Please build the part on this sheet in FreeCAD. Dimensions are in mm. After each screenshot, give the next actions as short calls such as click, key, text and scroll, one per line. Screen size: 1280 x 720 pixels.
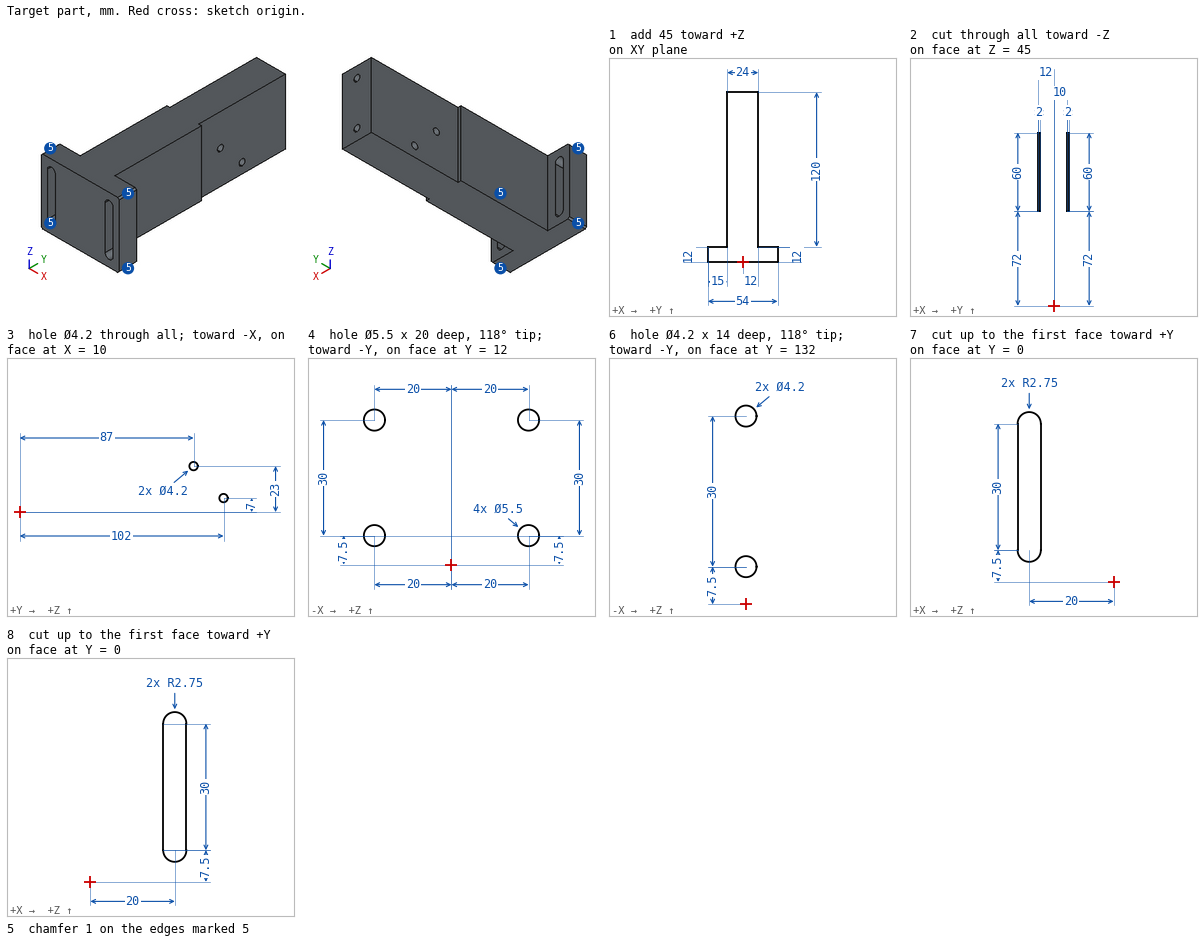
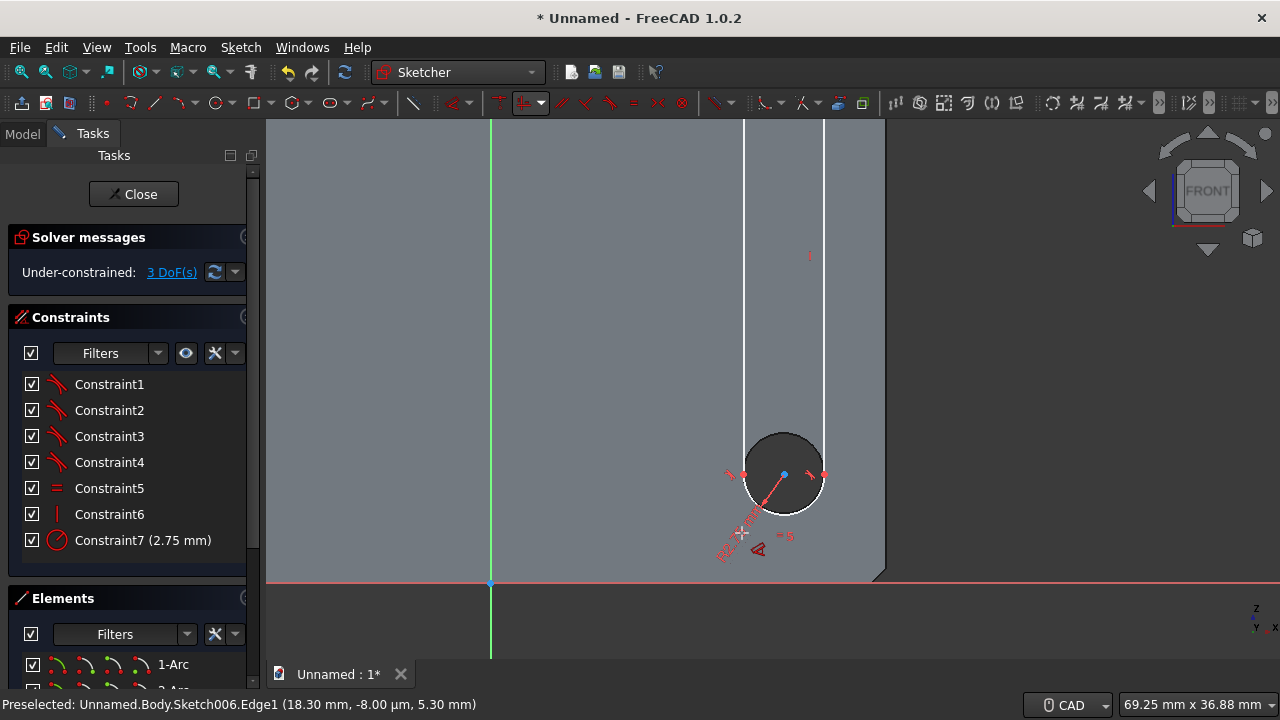
click(744, 343)
click(778, 311)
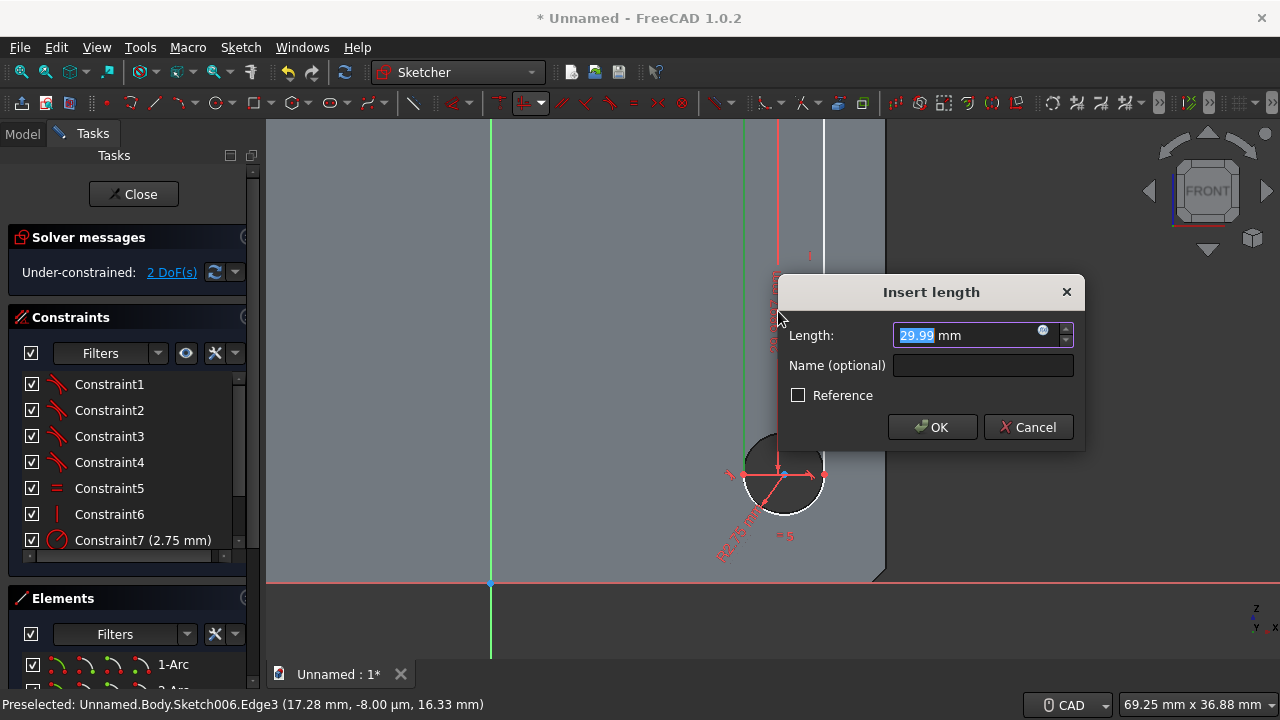
text(30)
key(Return)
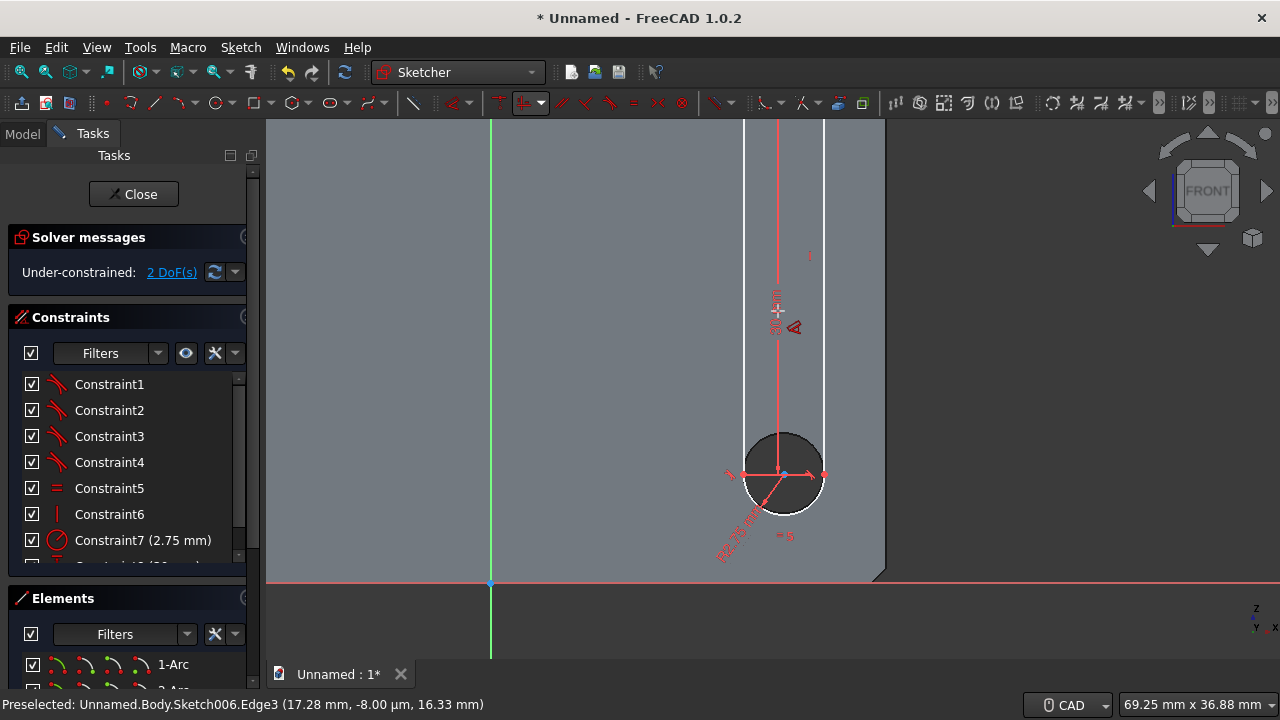
click(784, 475)
click(637, 617)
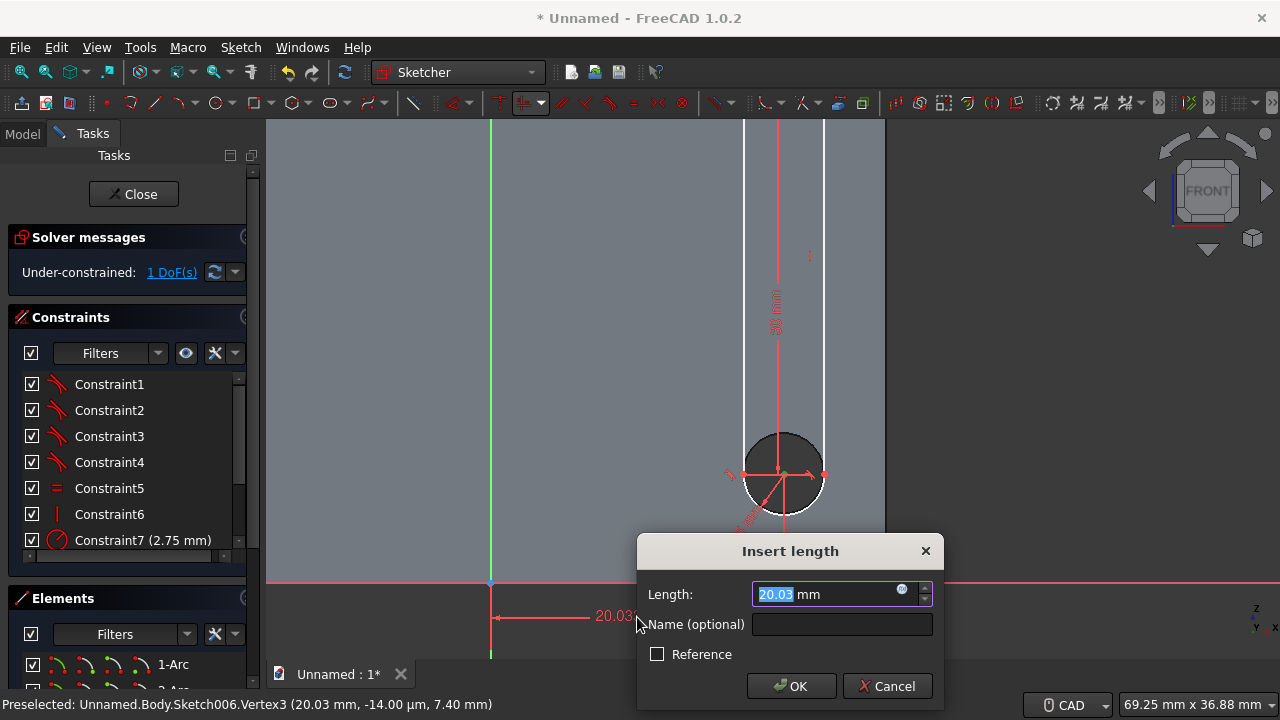
text(20)
key(Return)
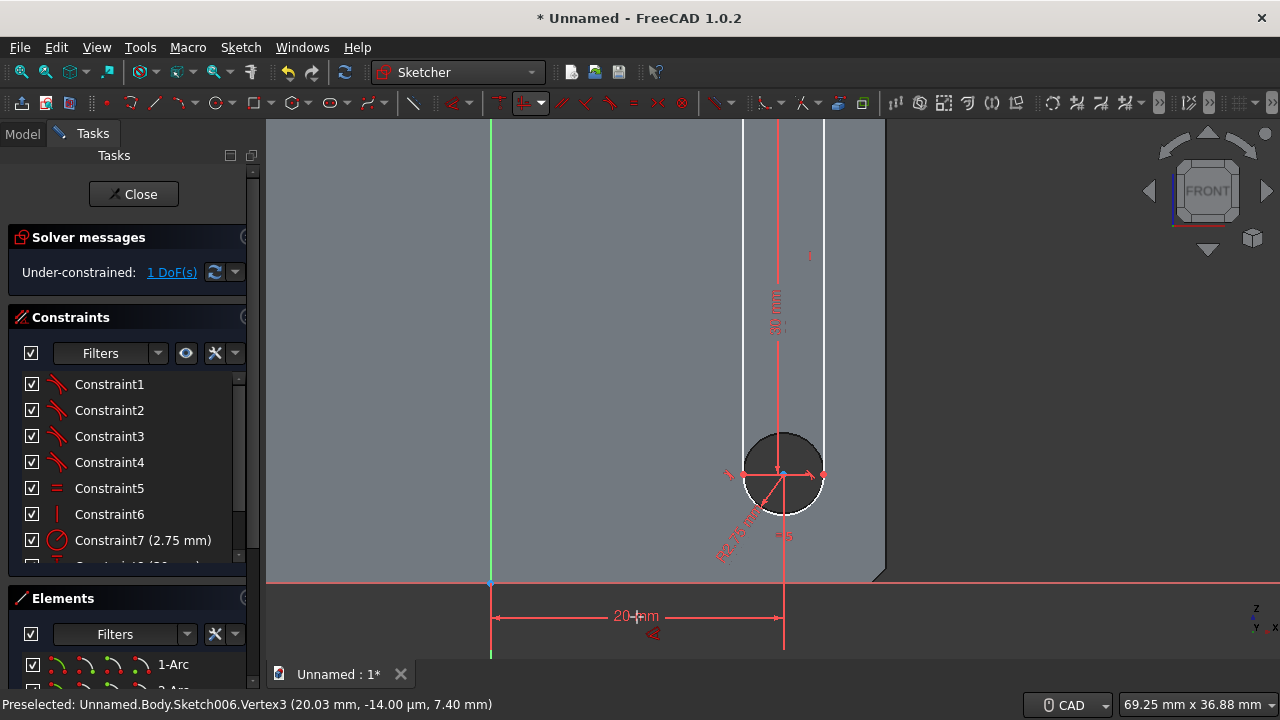
click(743, 475)
click(457, 529)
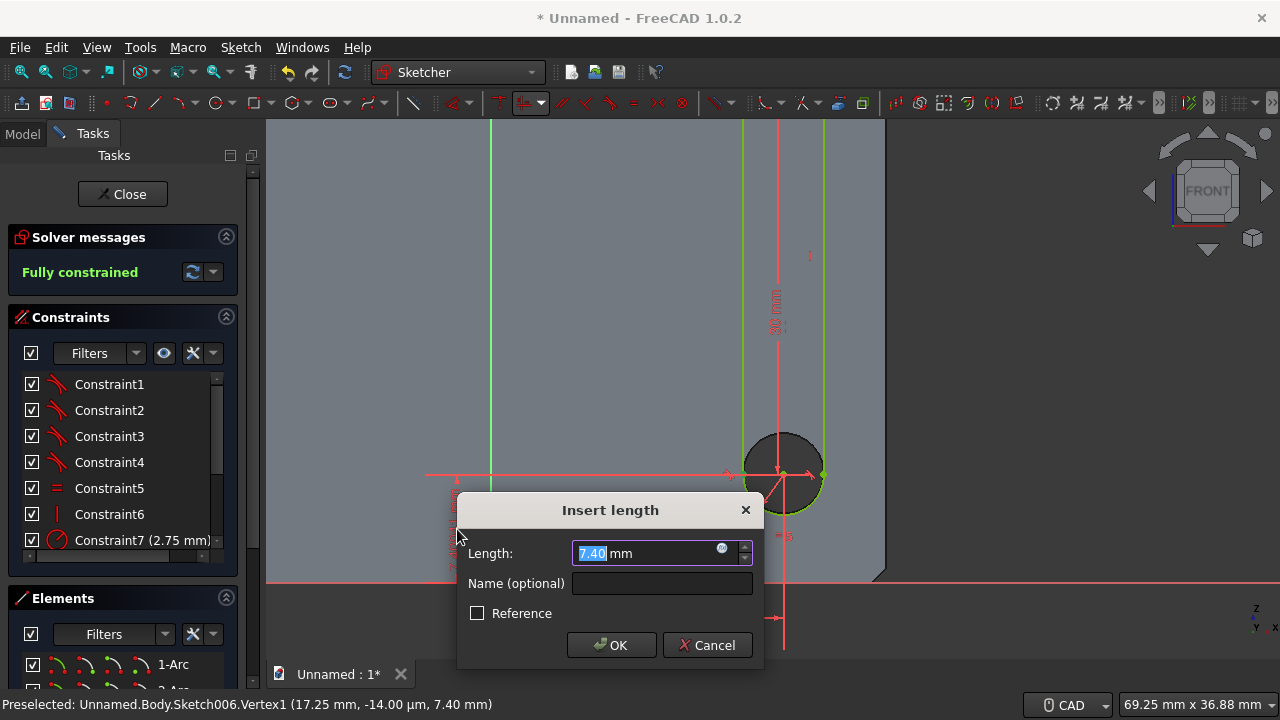
text(7.5)
key(Return)
key(Escape)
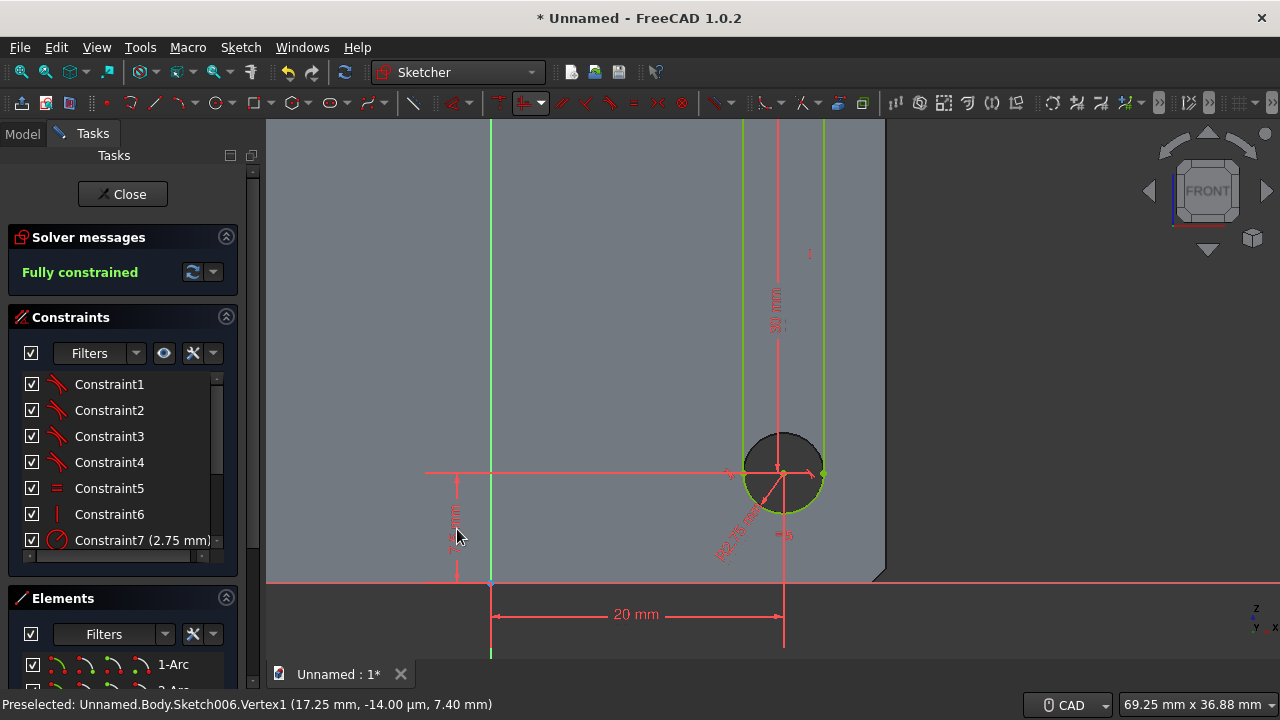
click(123, 194)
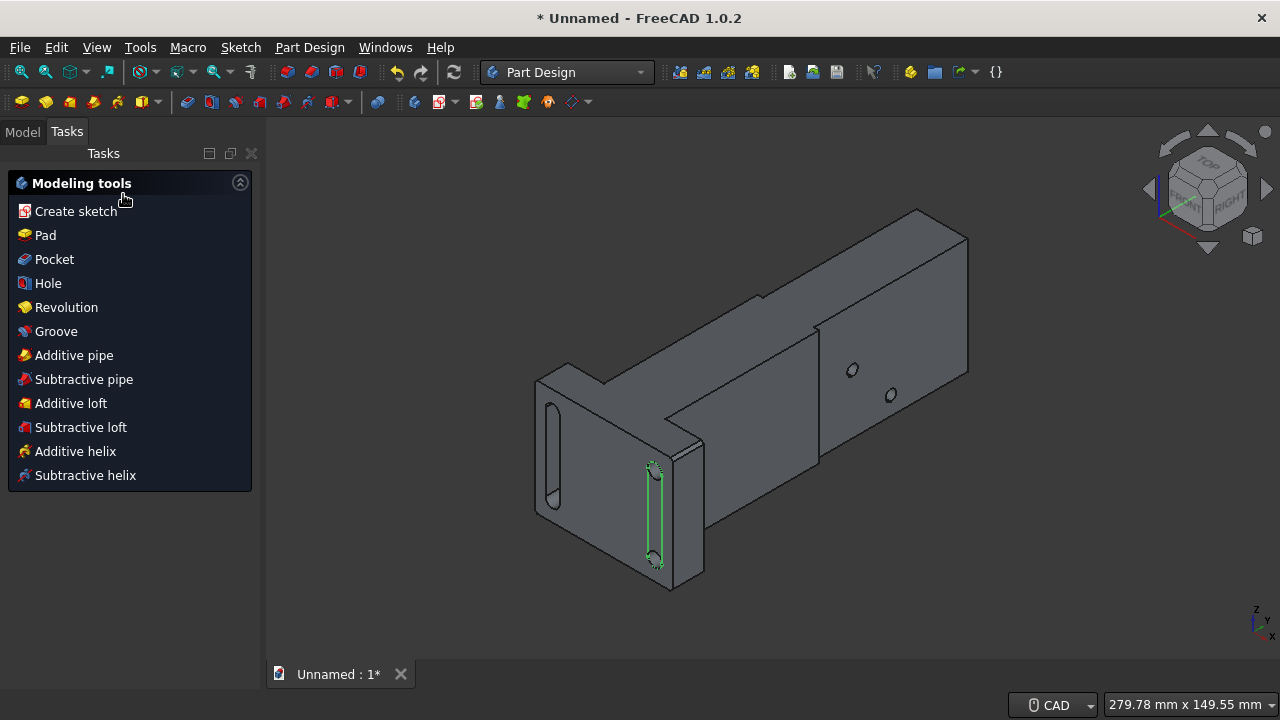
click(188, 102)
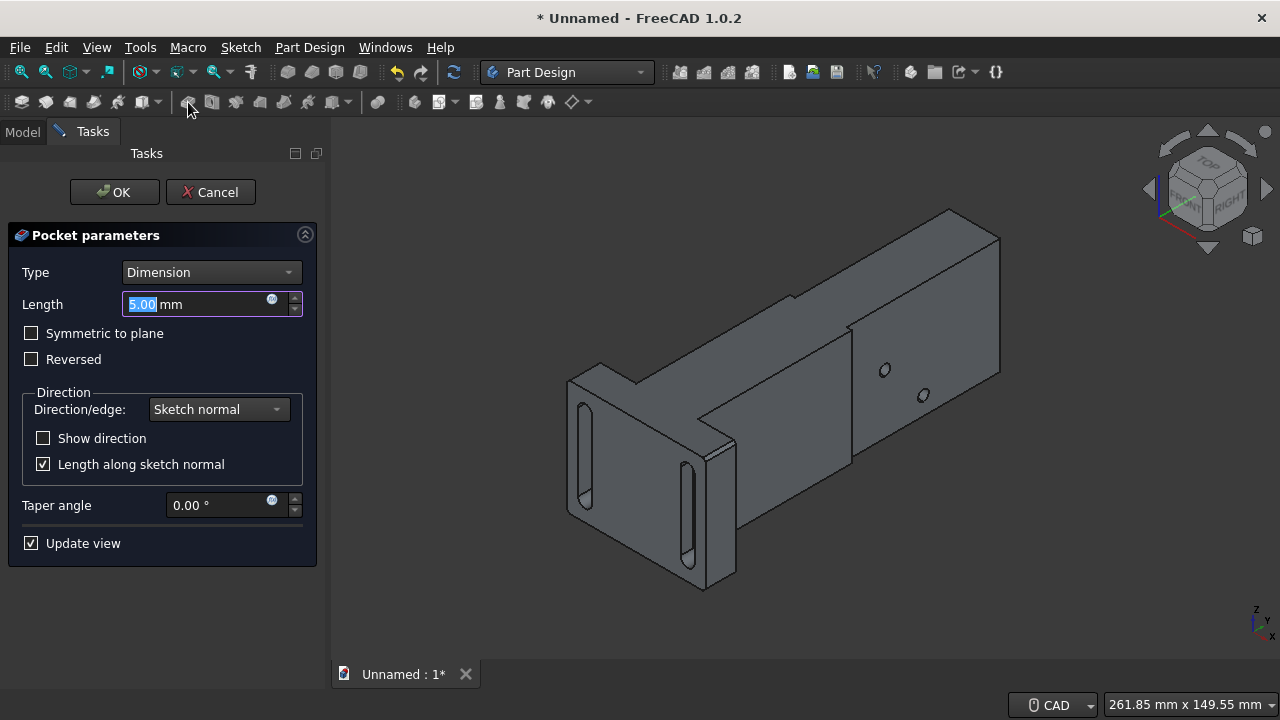
click(212, 272)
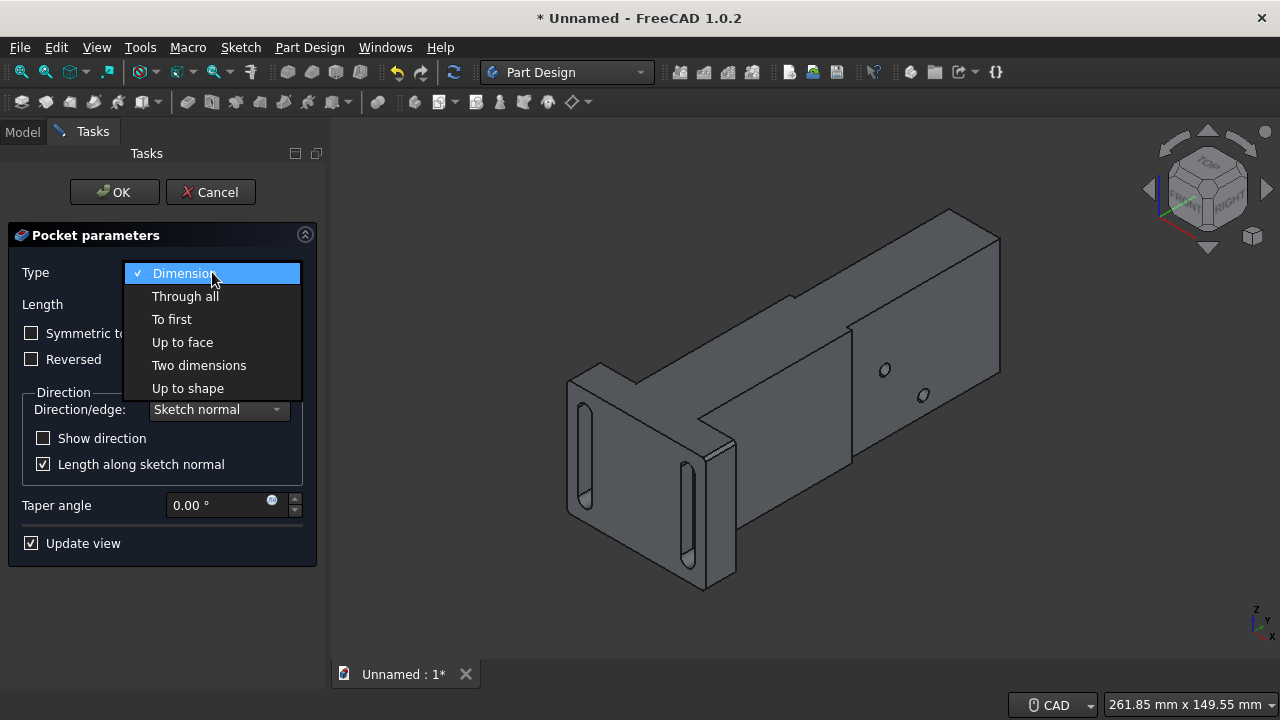
click(212, 320)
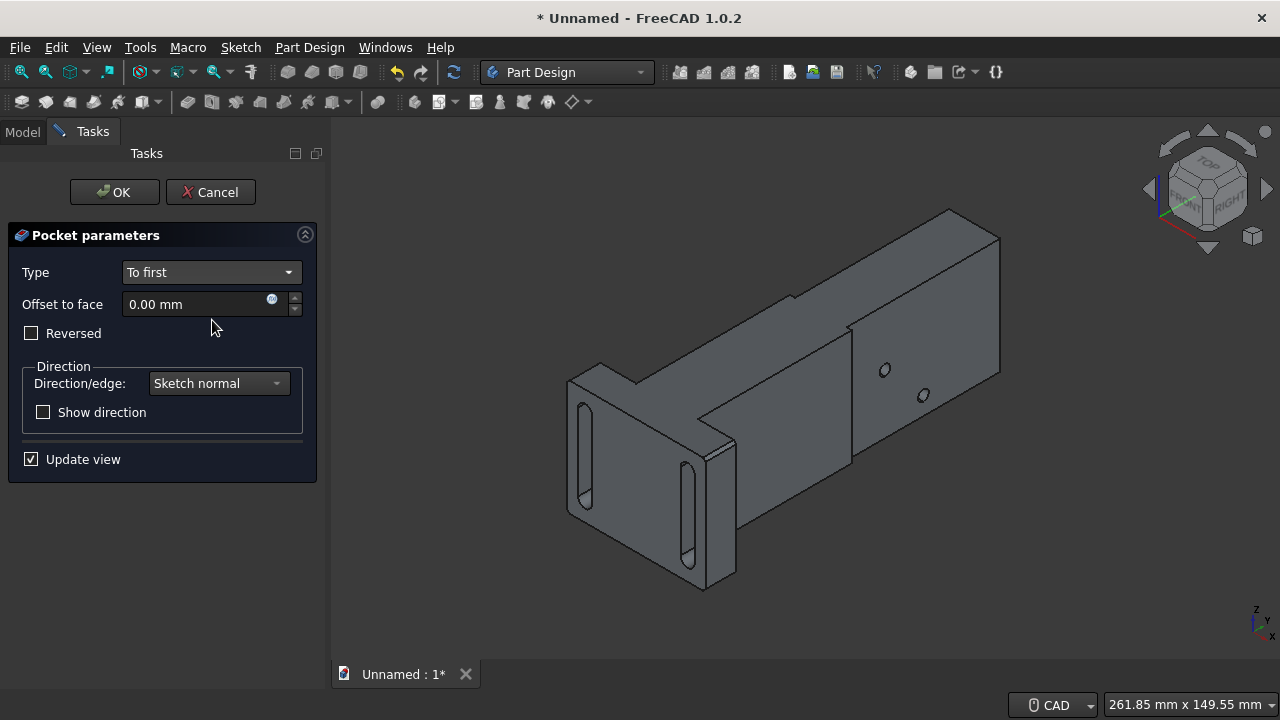
click(115, 192)